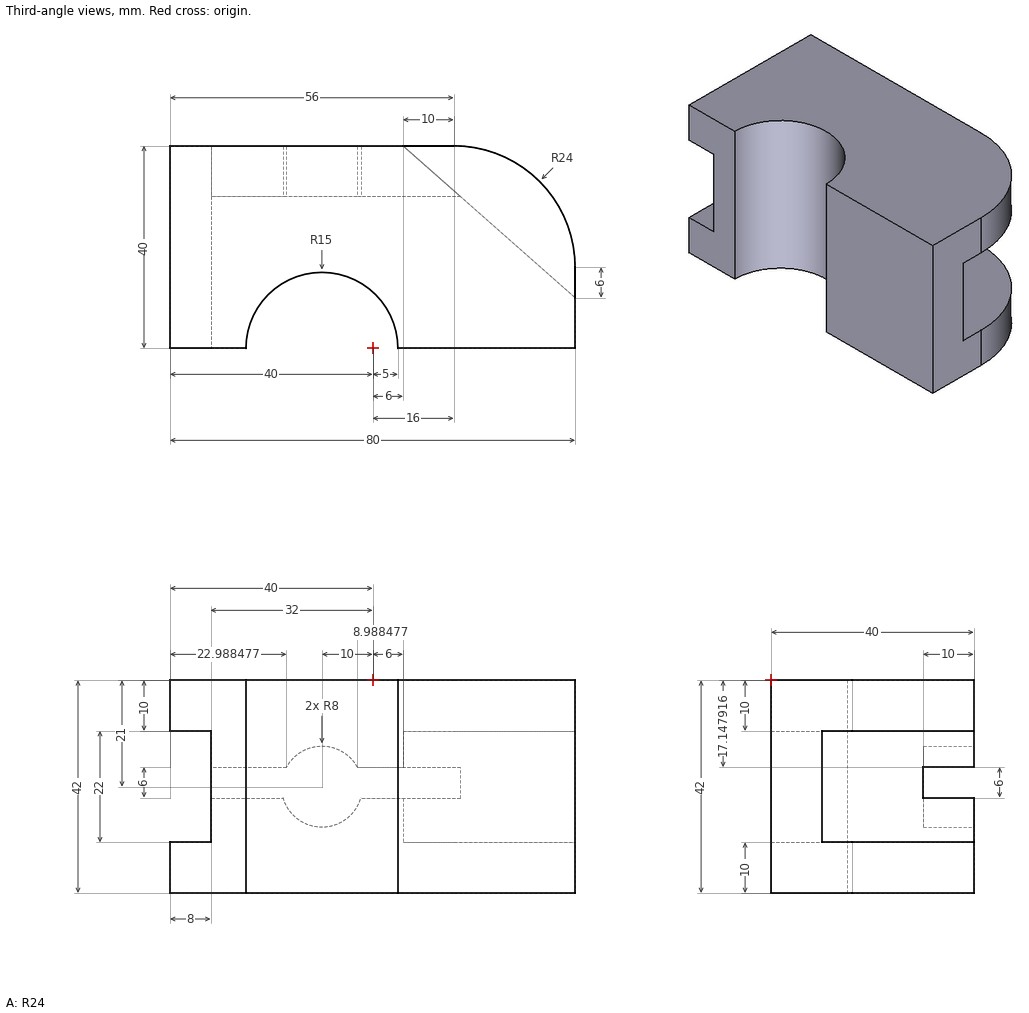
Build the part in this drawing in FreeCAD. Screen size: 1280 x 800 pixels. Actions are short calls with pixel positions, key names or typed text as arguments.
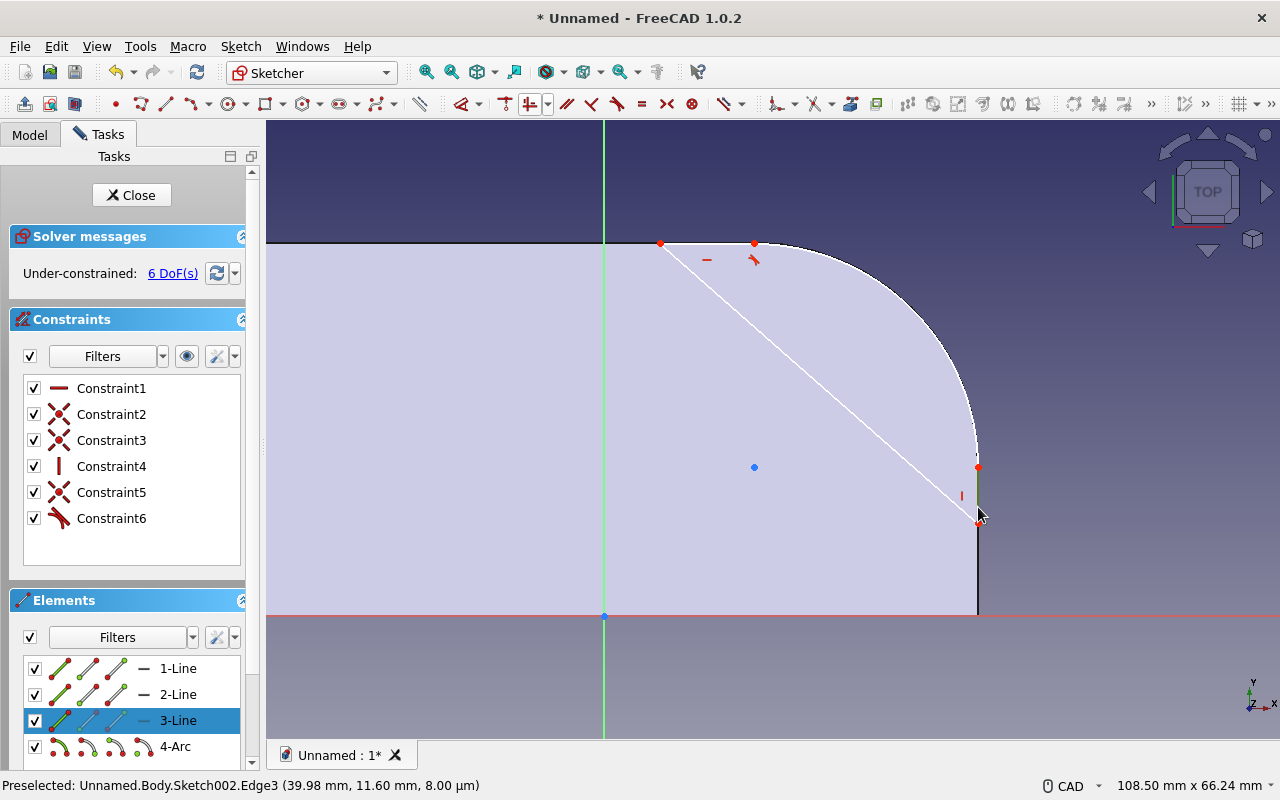
click(954, 366)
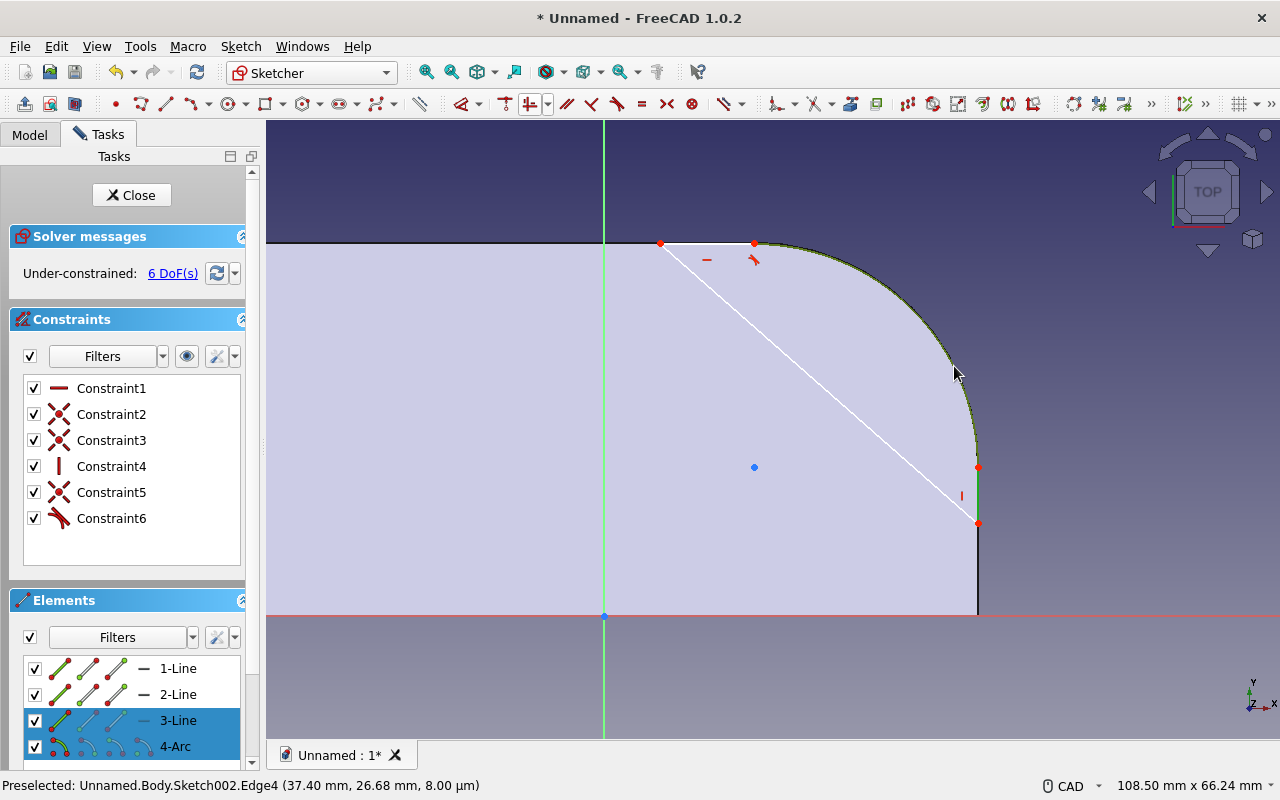
key(t)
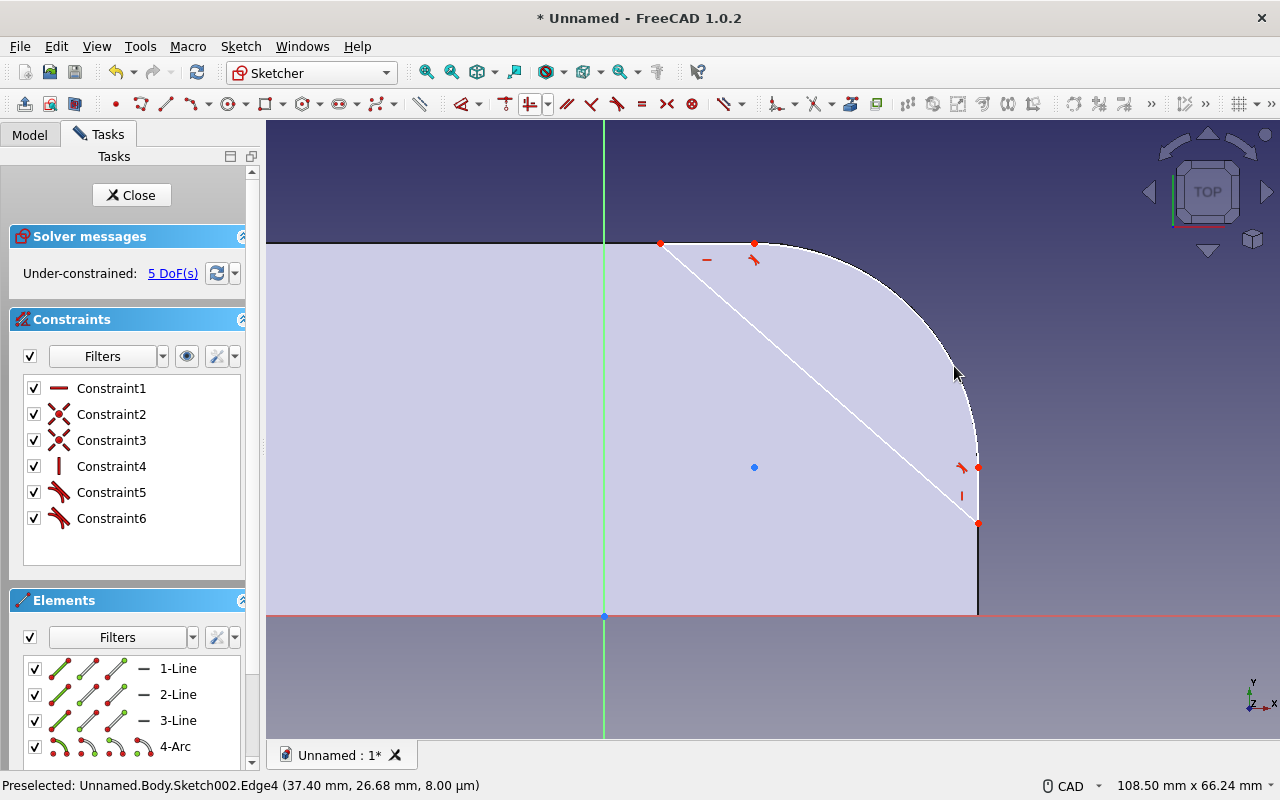
key(d)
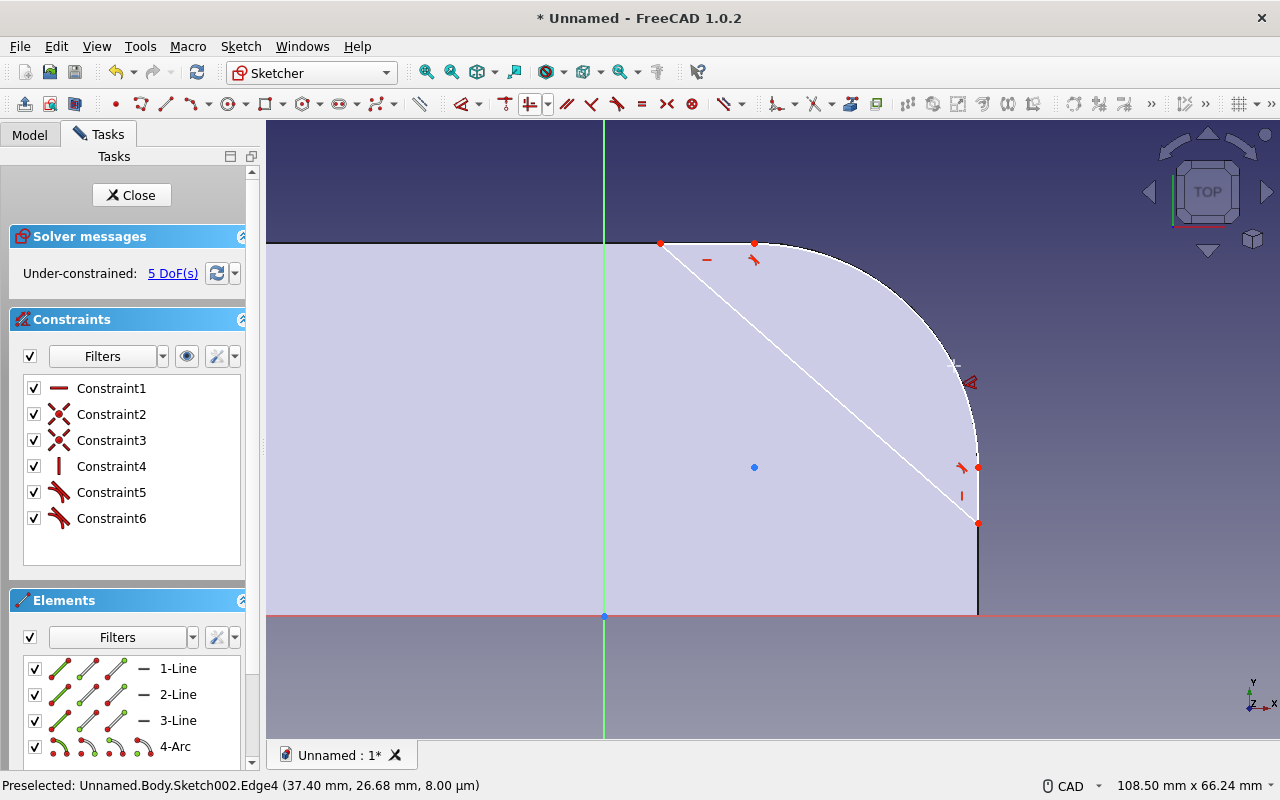
click(954, 366)
click(983, 351)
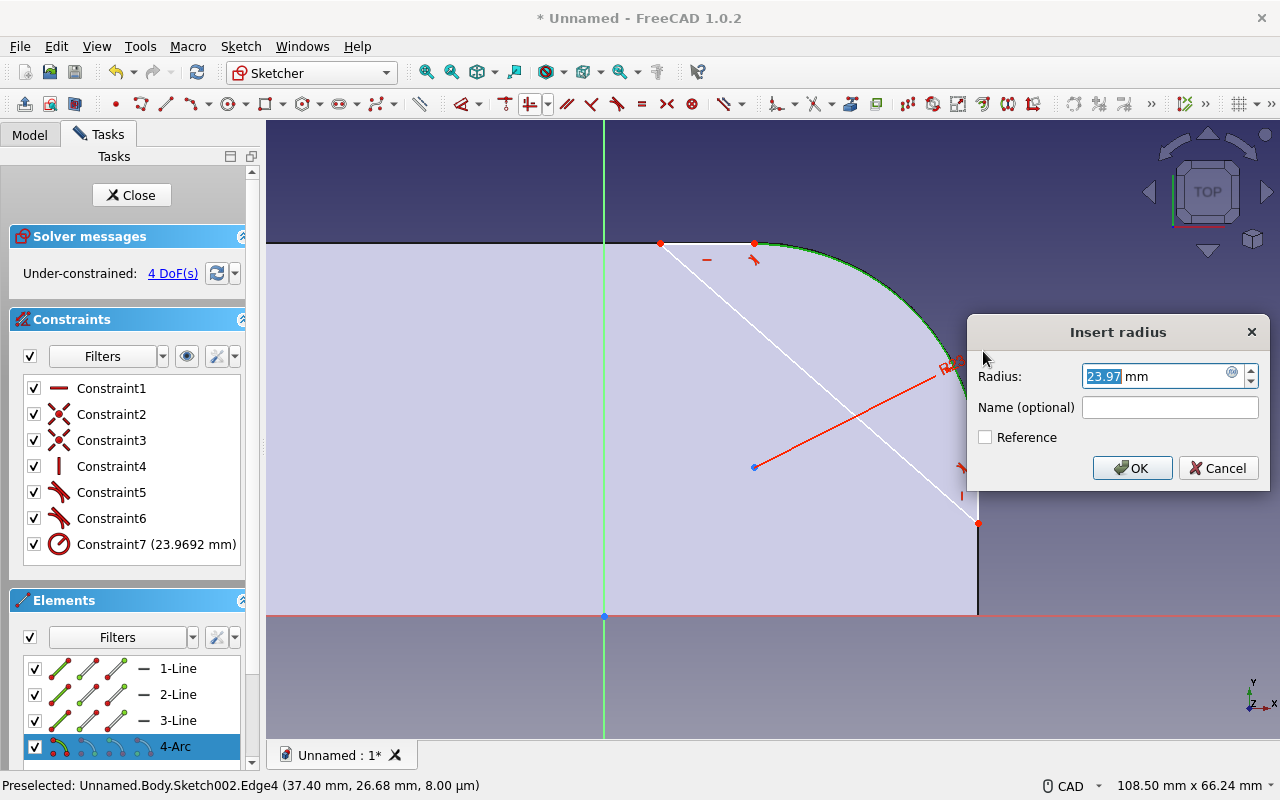
text(24)
key(Return)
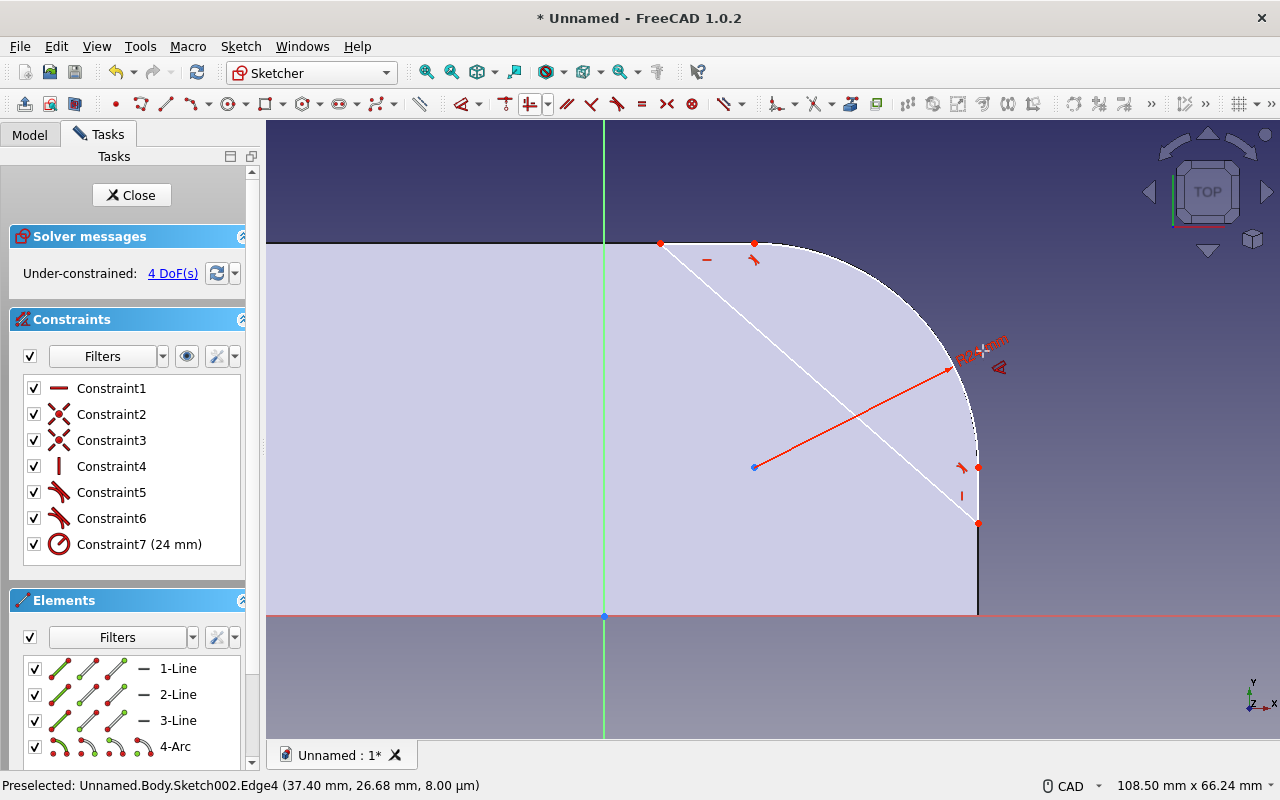
click(978, 507)
click(1012, 496)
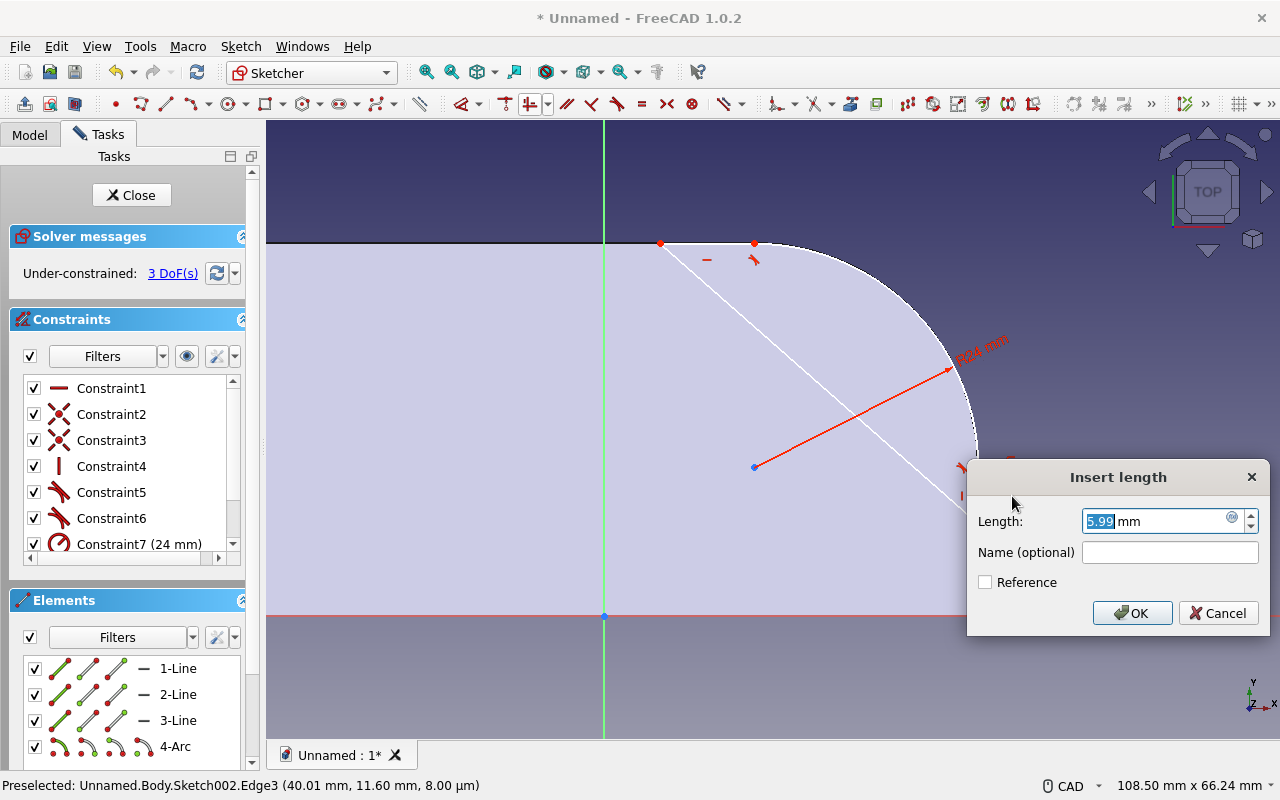
text(6)
key(Return)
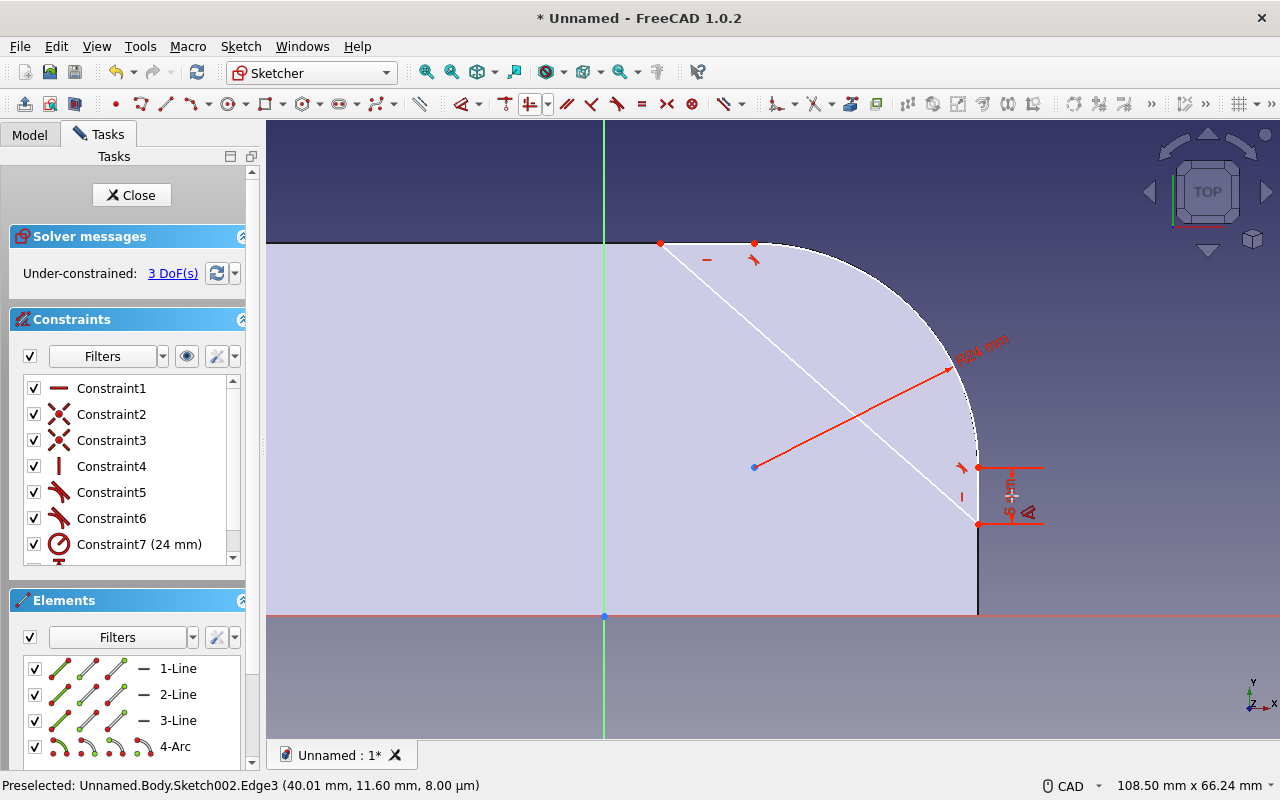
click(726, 244)
click(707, 210)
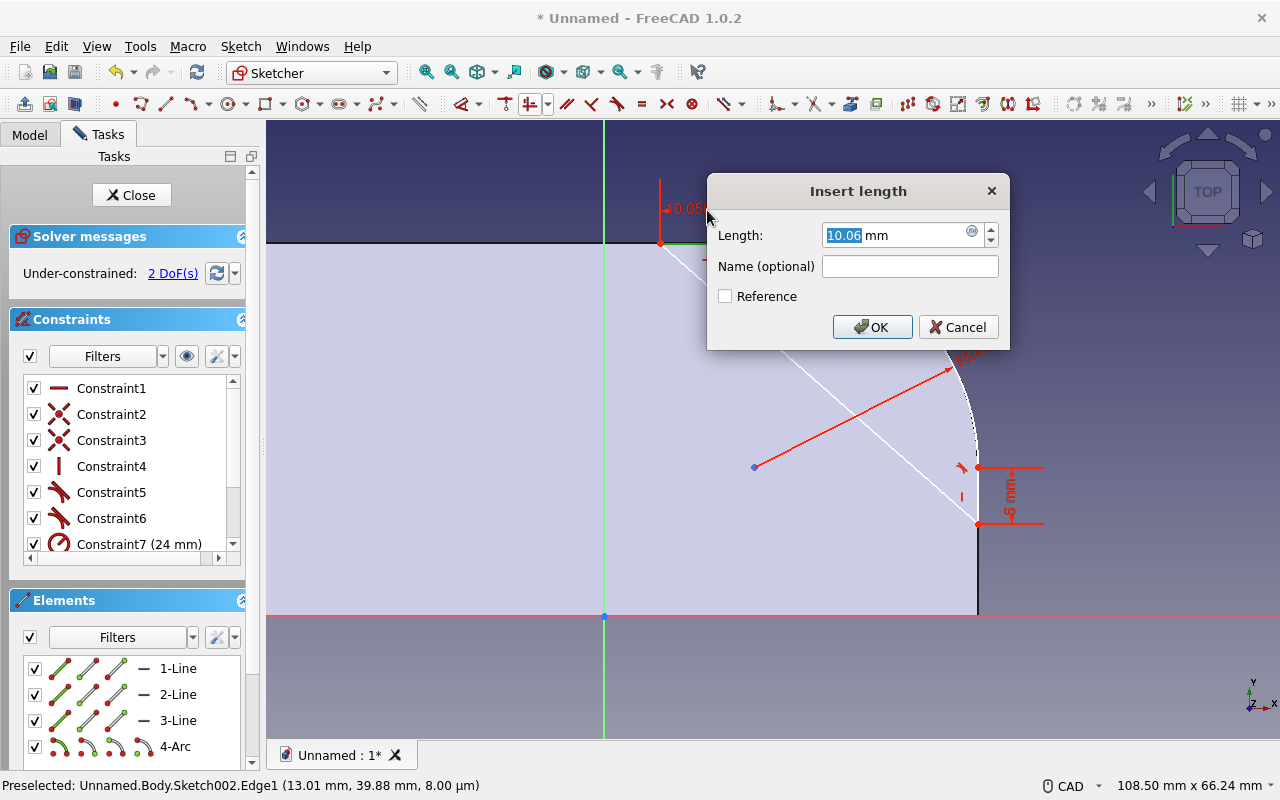
text(10)
key(Return)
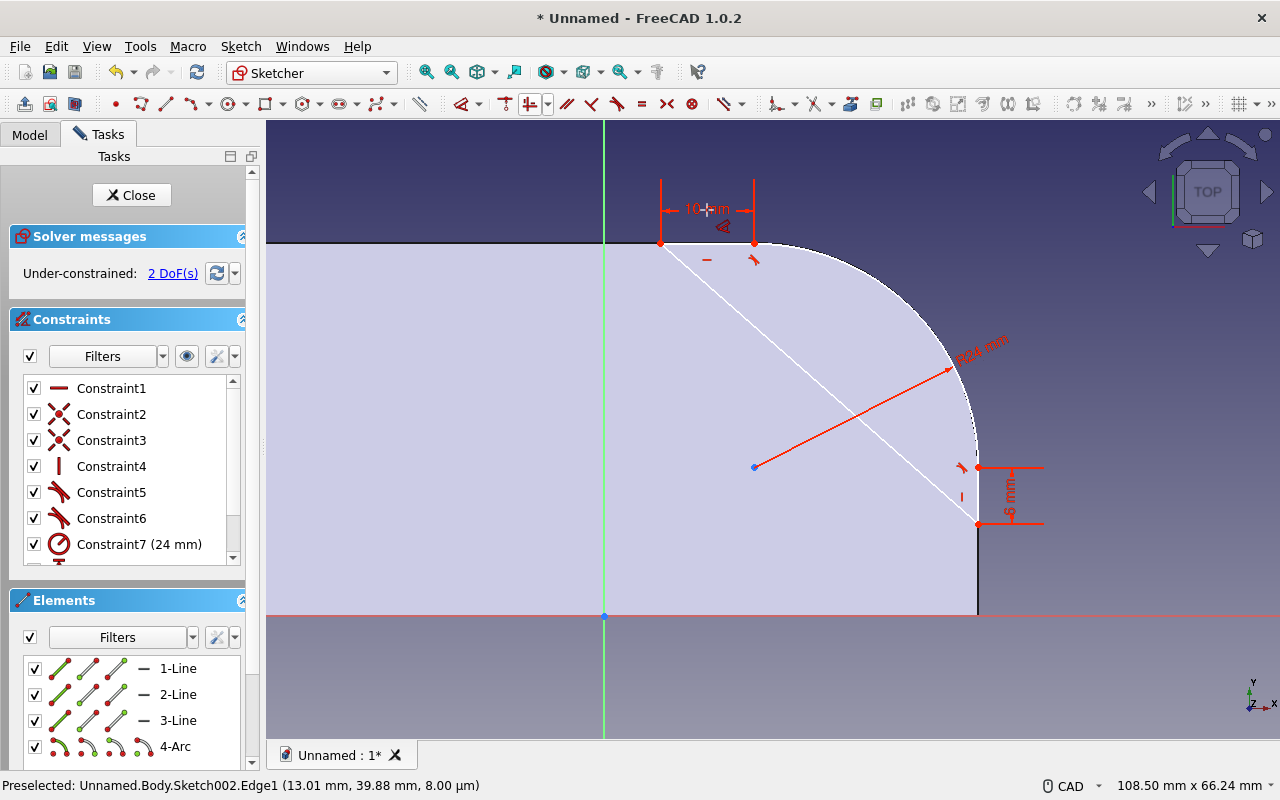
click(661, 244)
click(632, 650)